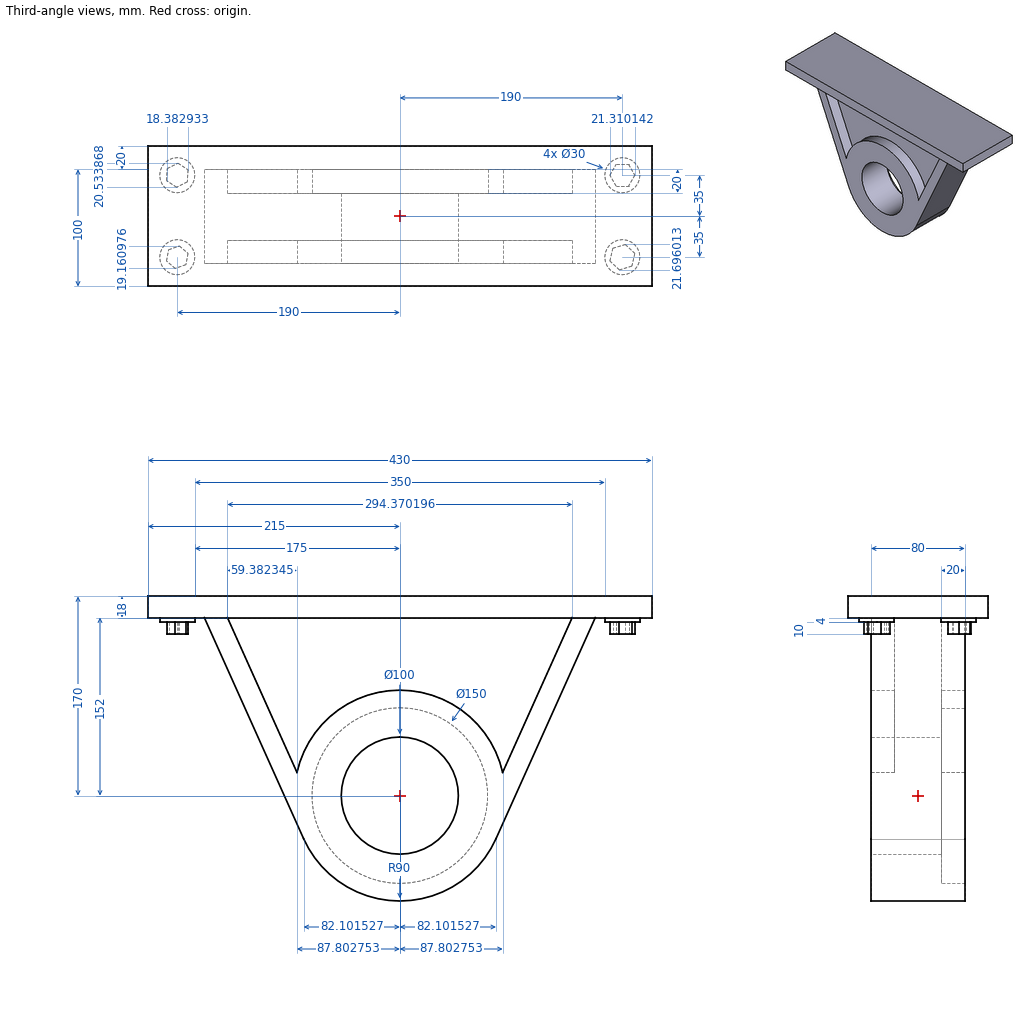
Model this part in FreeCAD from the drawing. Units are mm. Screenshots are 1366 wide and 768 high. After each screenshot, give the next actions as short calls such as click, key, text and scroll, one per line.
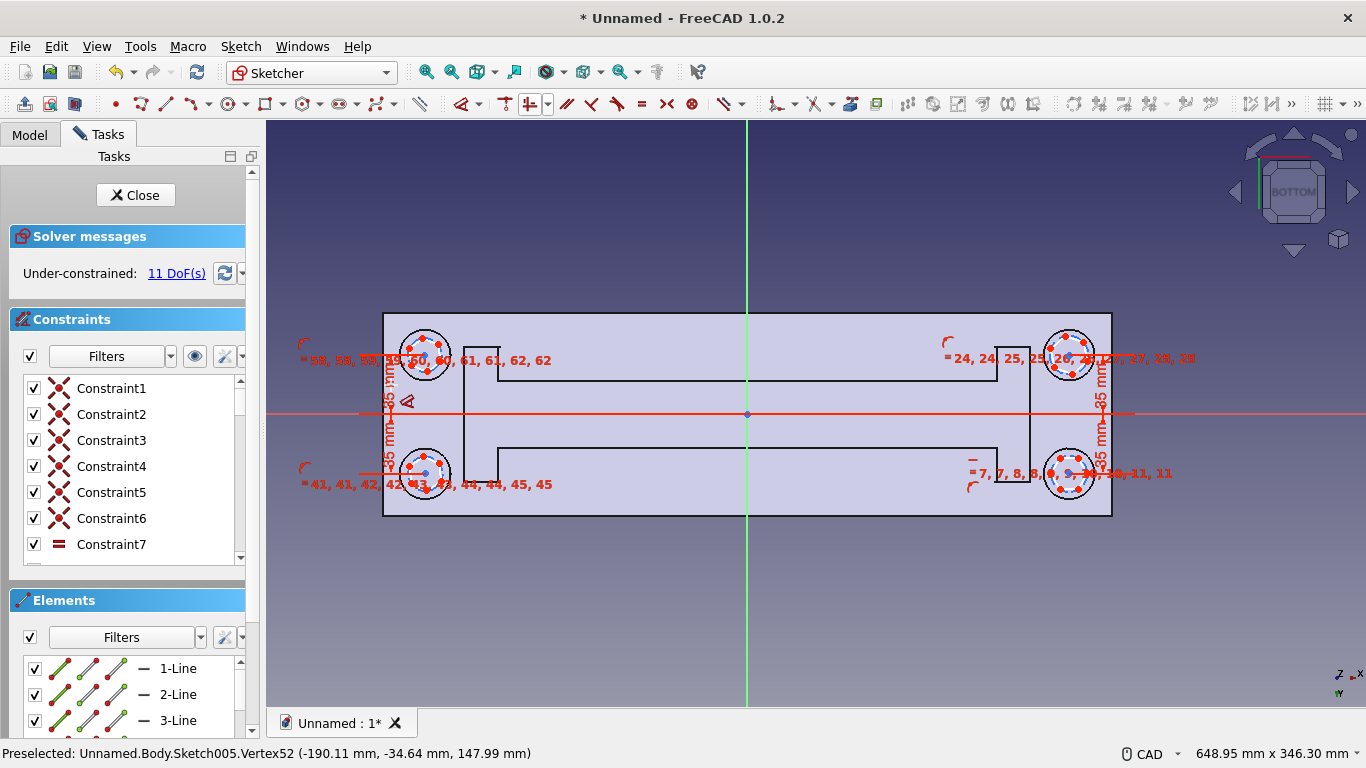
click(1069, 474)
click(908, 508)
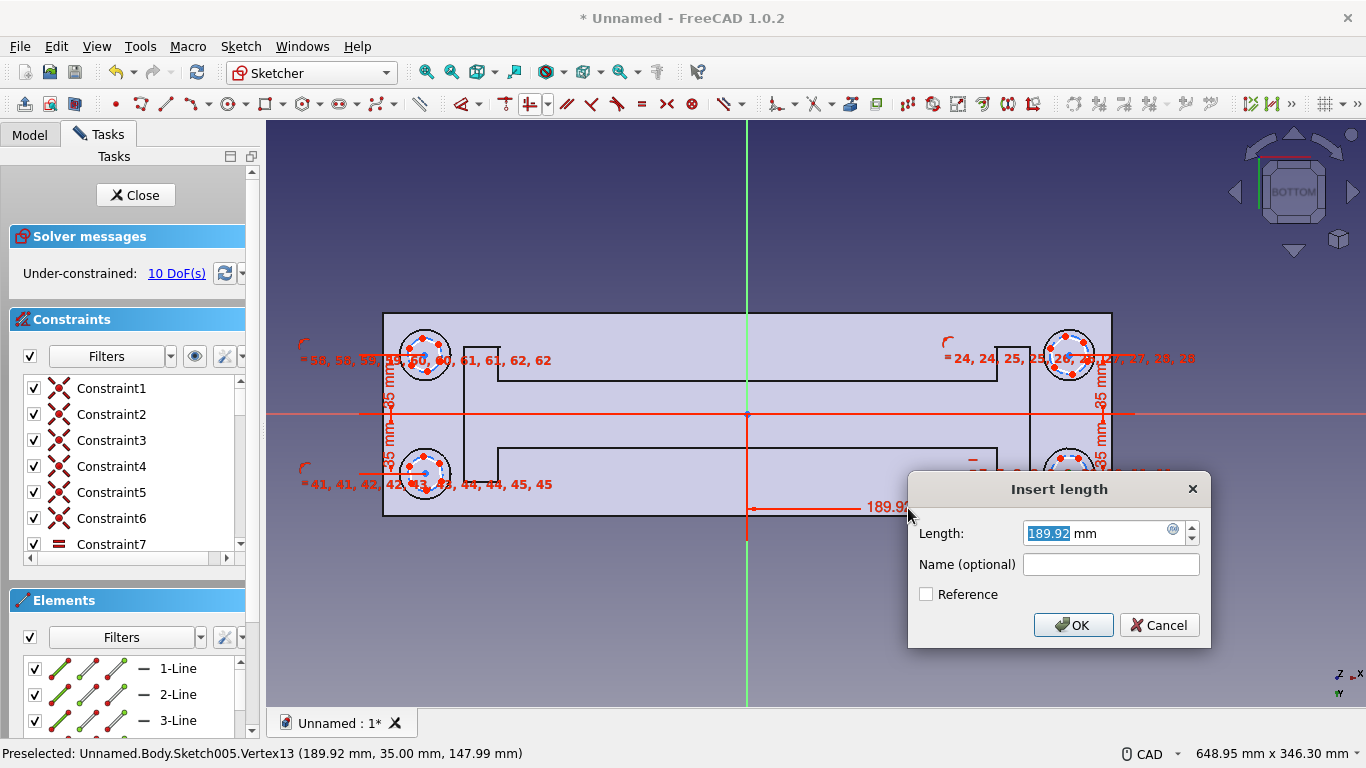
text(190)
key(Return)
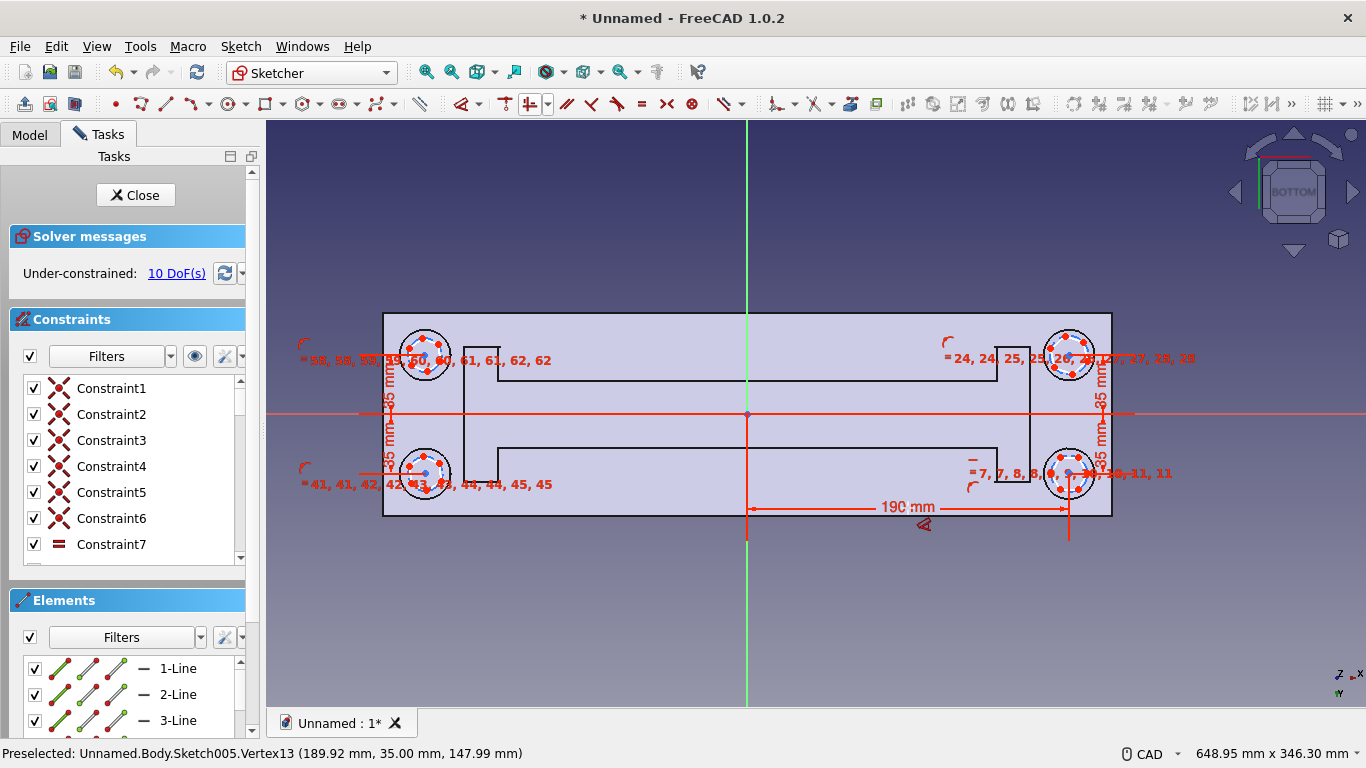
click(1069, 355)
click(908, 321)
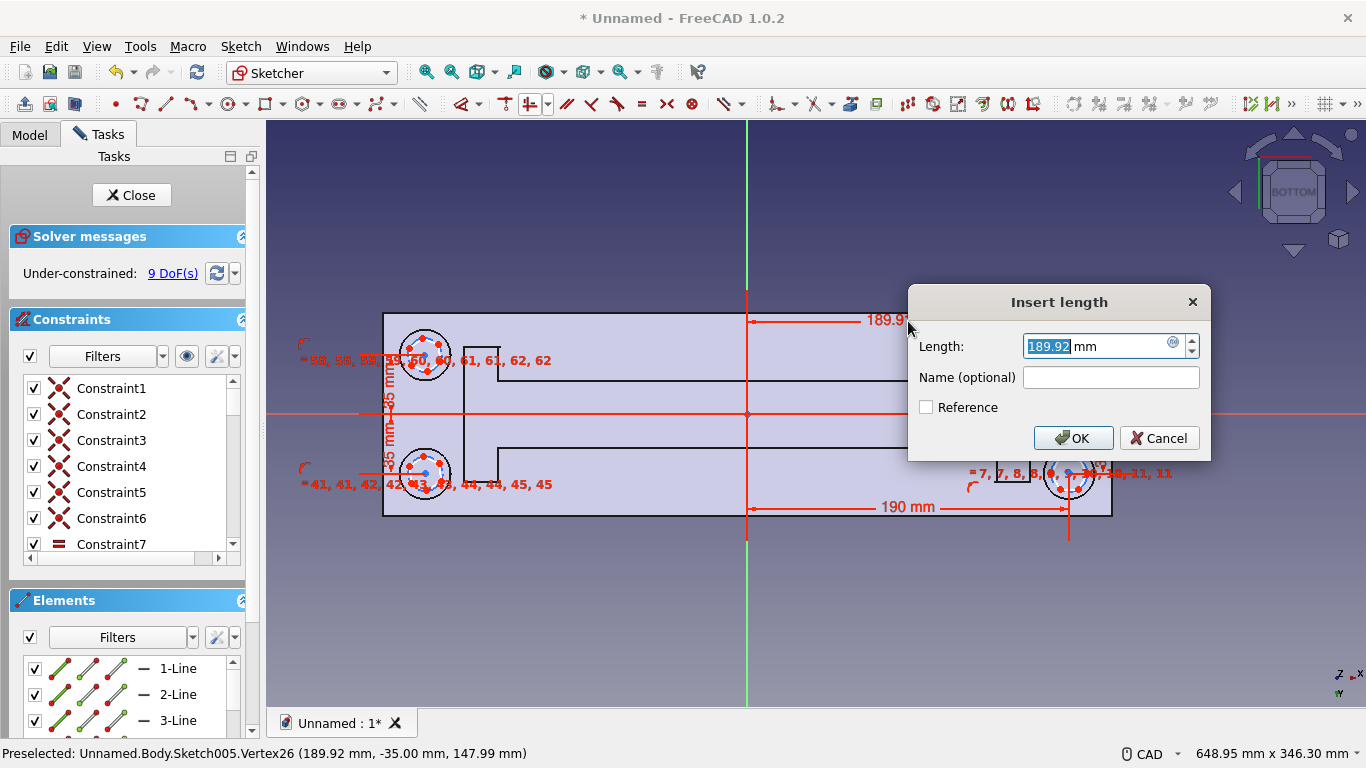
text(190)
key(Return)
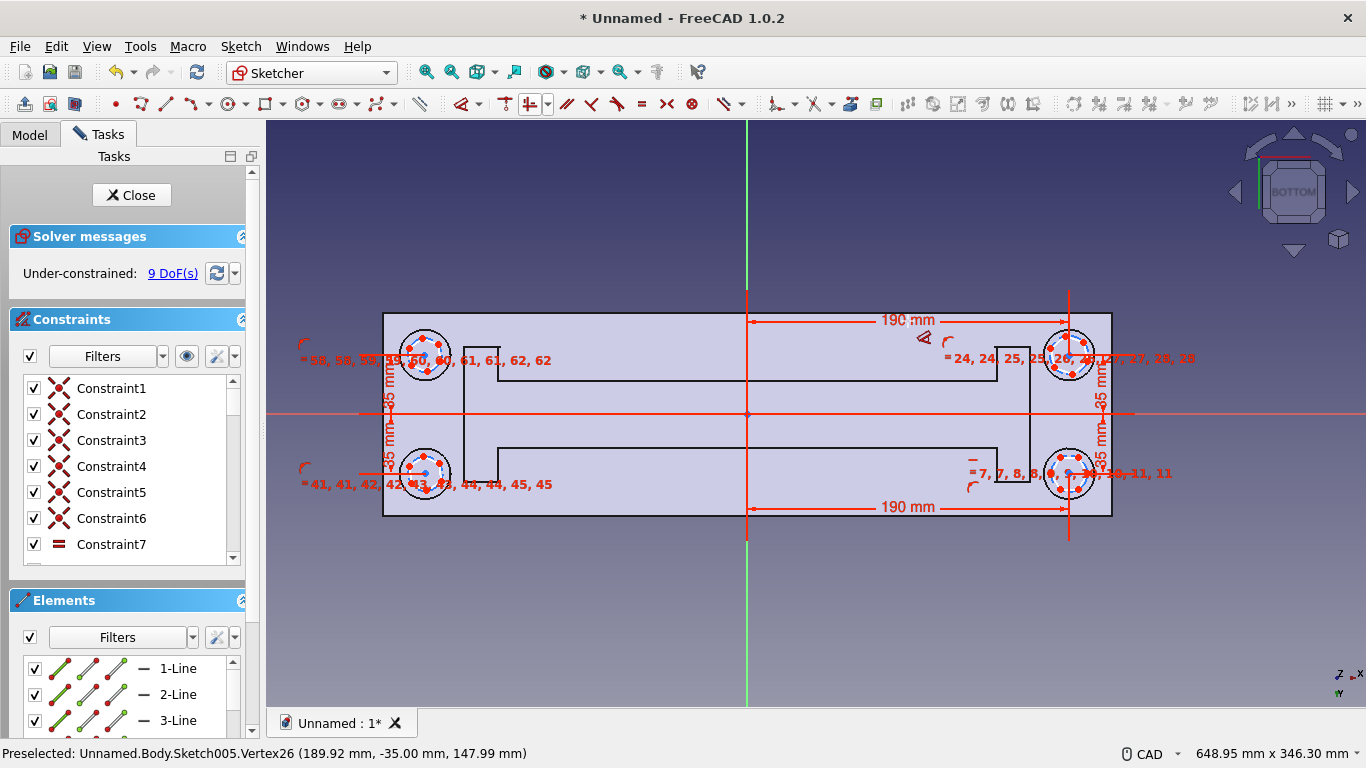
click(425, 474)
click(586, 508)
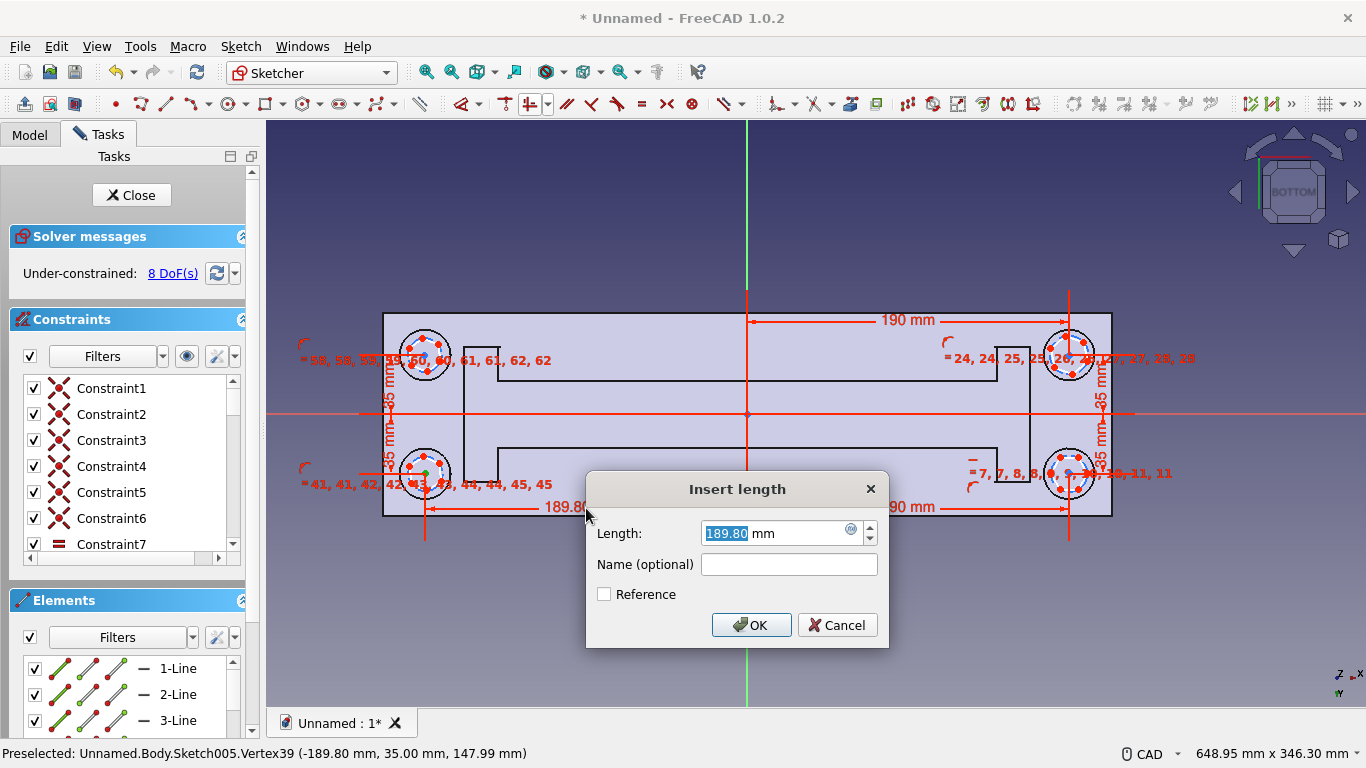
text(190)
key(Return)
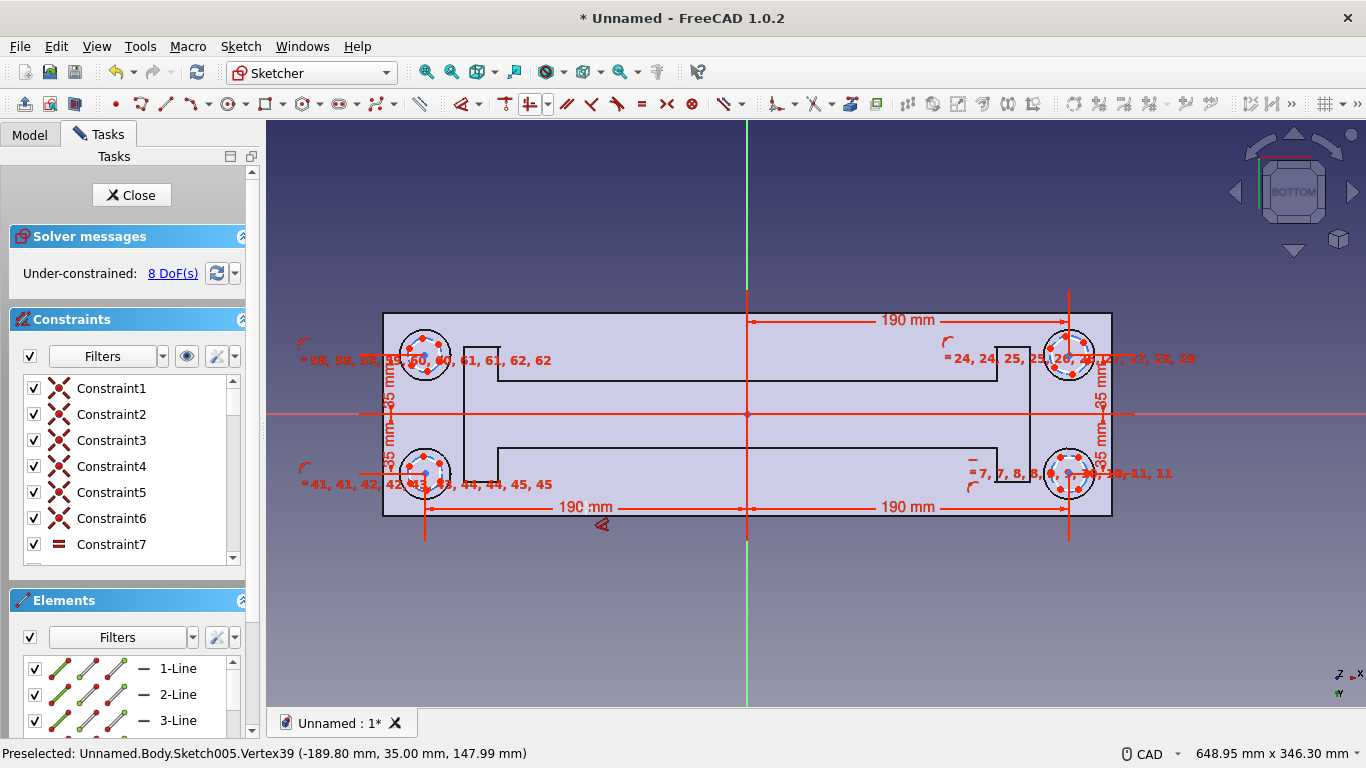
click(425, 355)
click(586, 321)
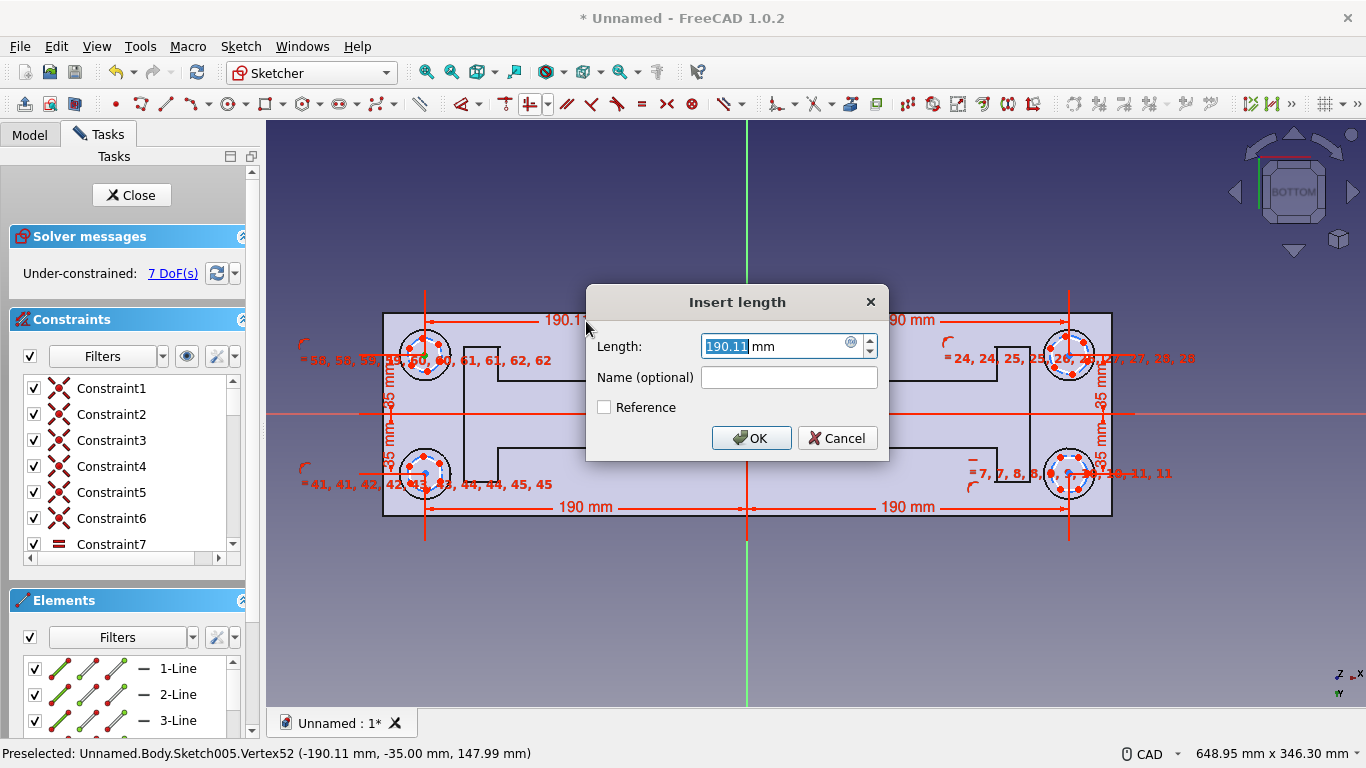
text(190)
key(Return)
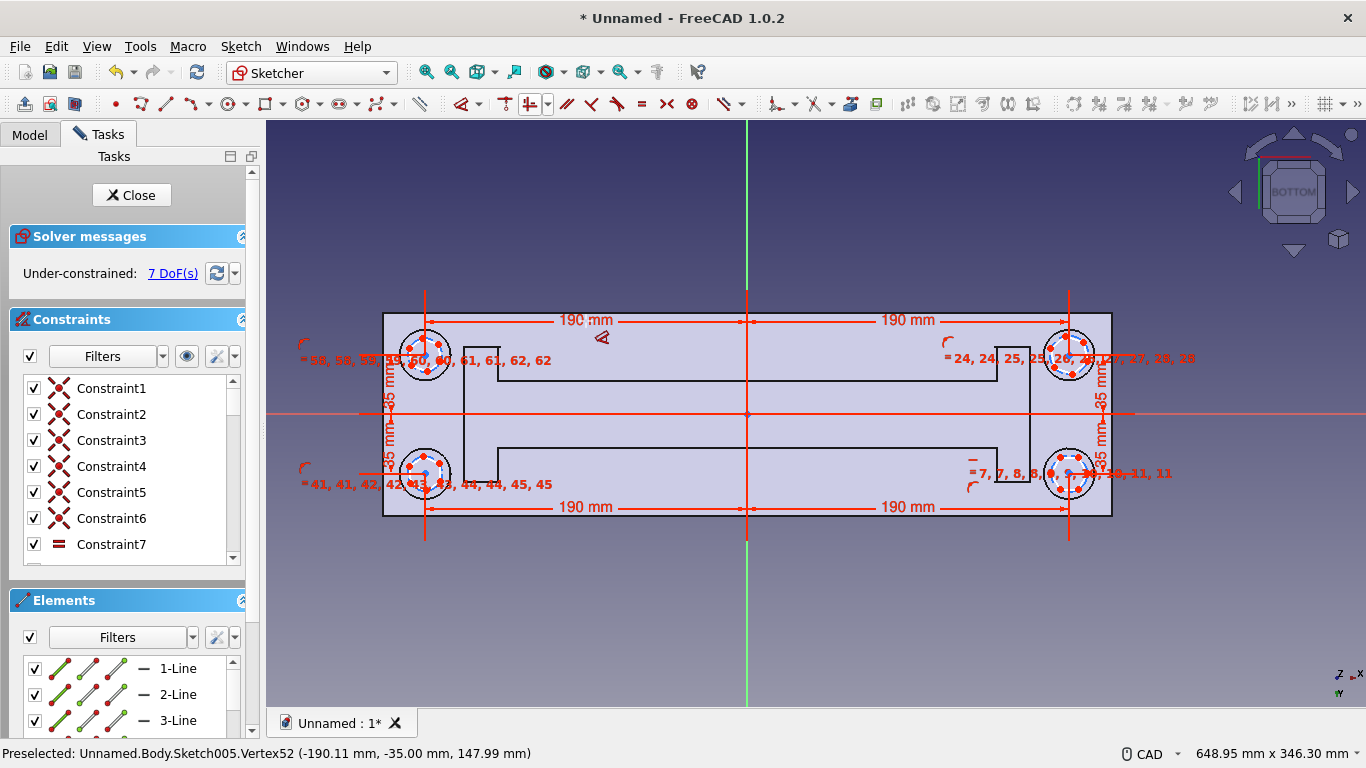
click(1051, 474)